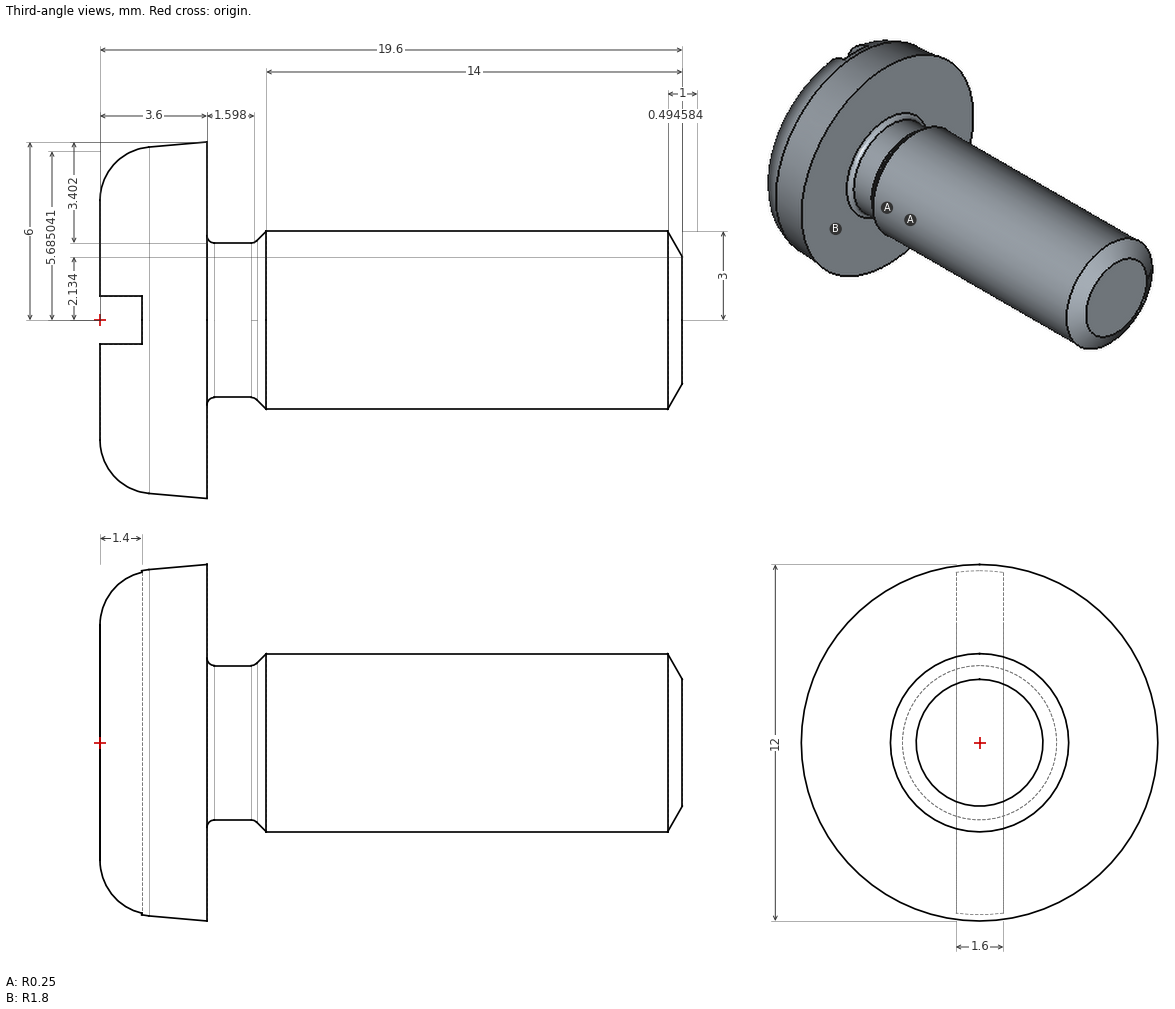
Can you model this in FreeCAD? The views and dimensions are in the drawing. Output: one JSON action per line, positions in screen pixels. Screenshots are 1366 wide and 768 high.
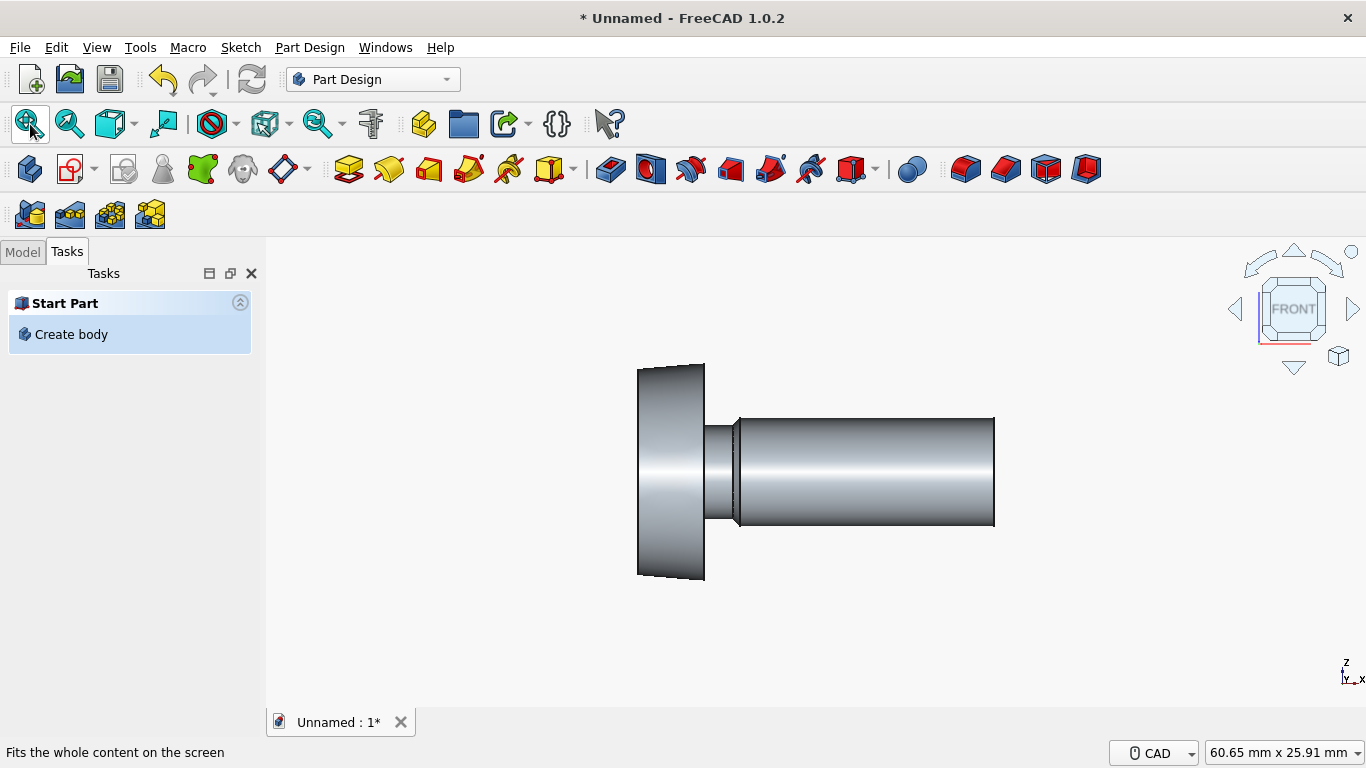
{"action": "key", "text": "3"}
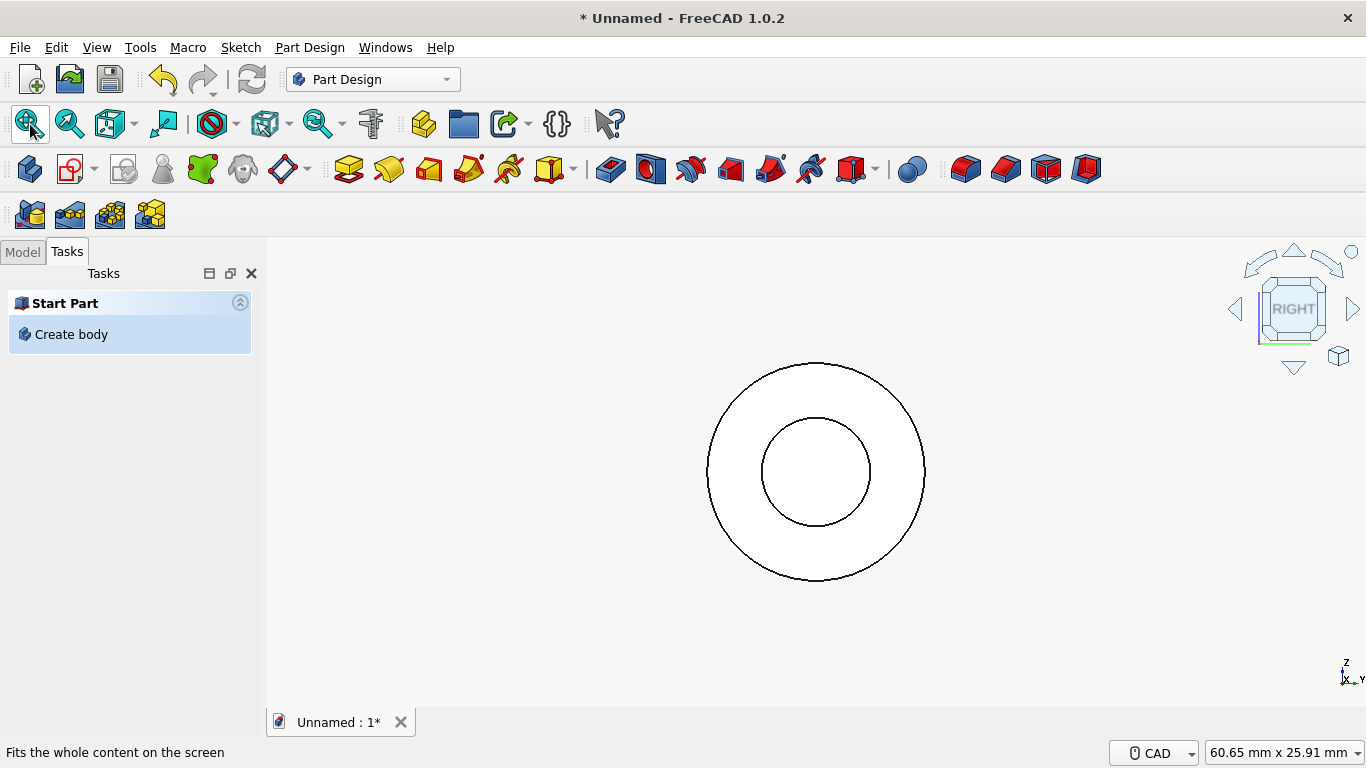
{"action": "key", "text": "5"}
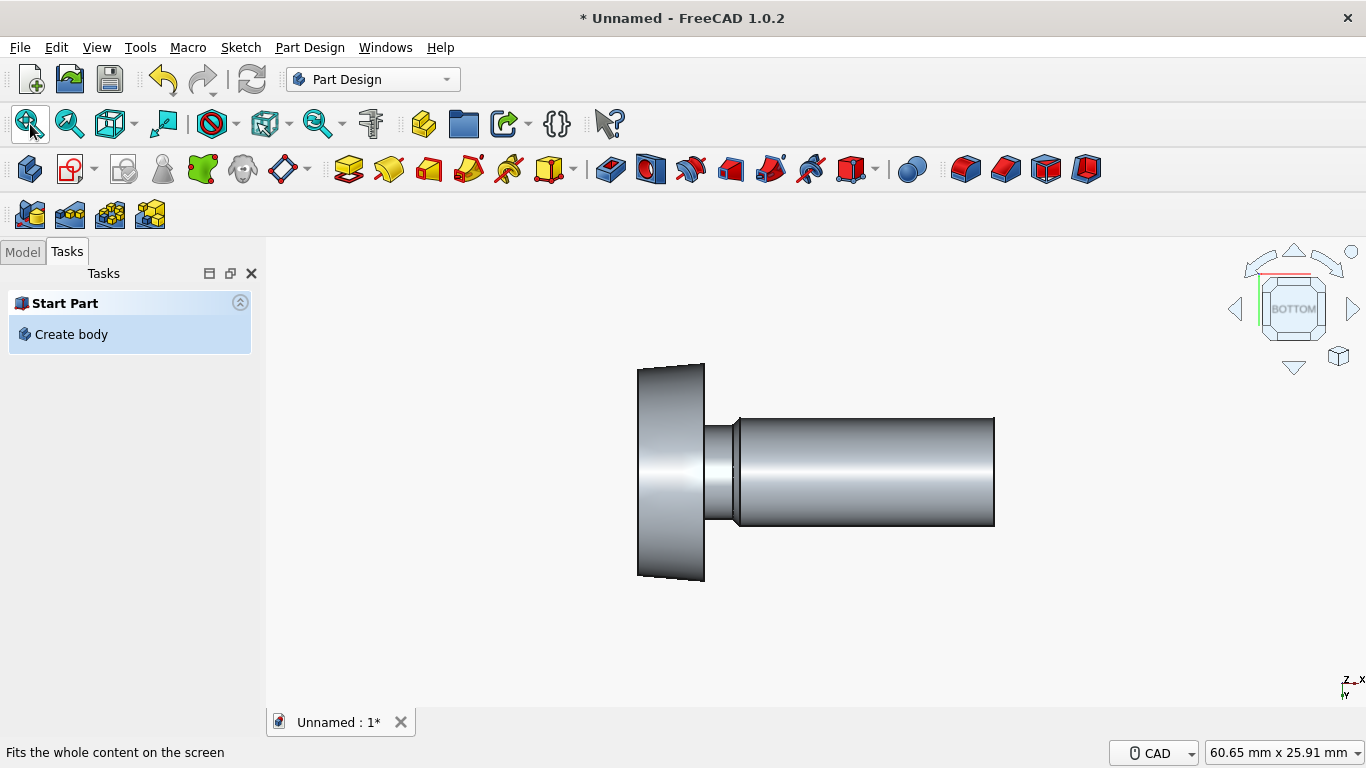
{"action": "key", "text": "4"}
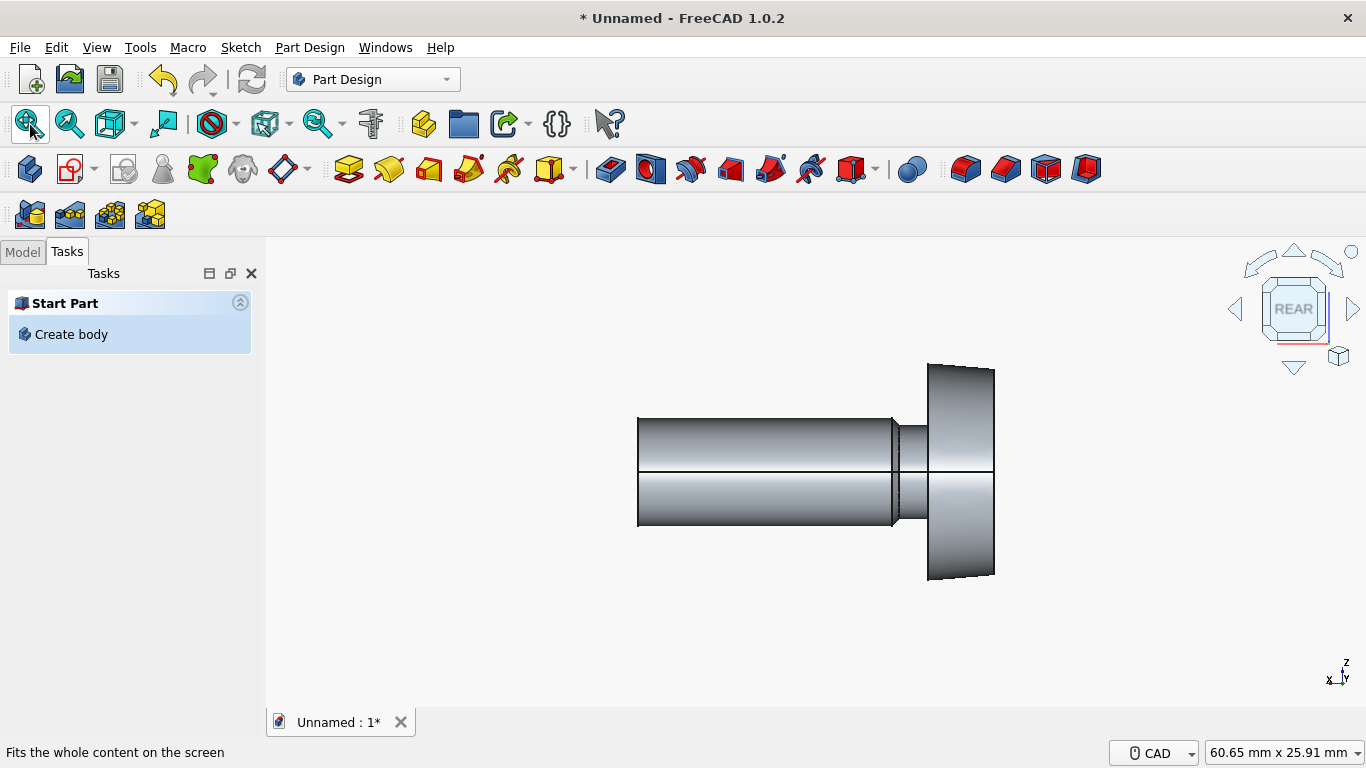
{"action": "key", "text": "6"}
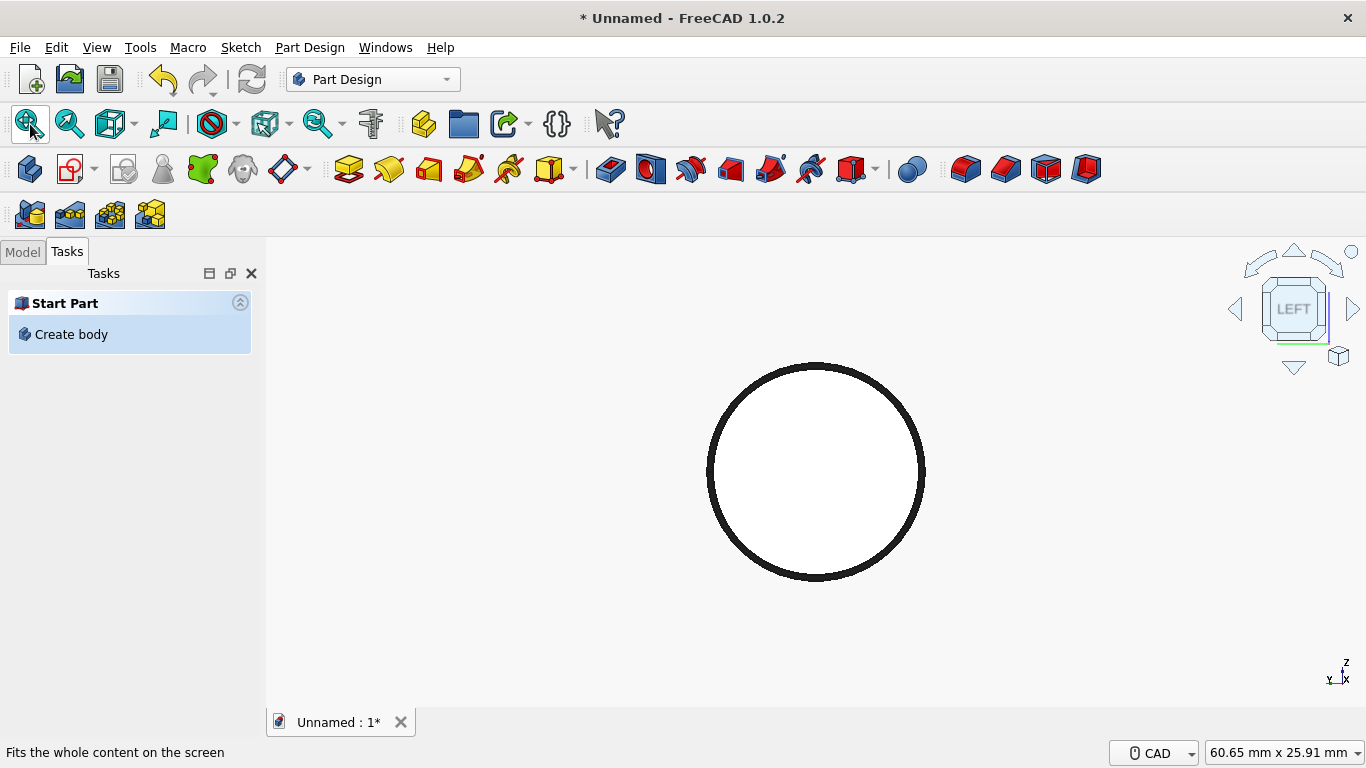
{"action": "key", "text": "v 3"}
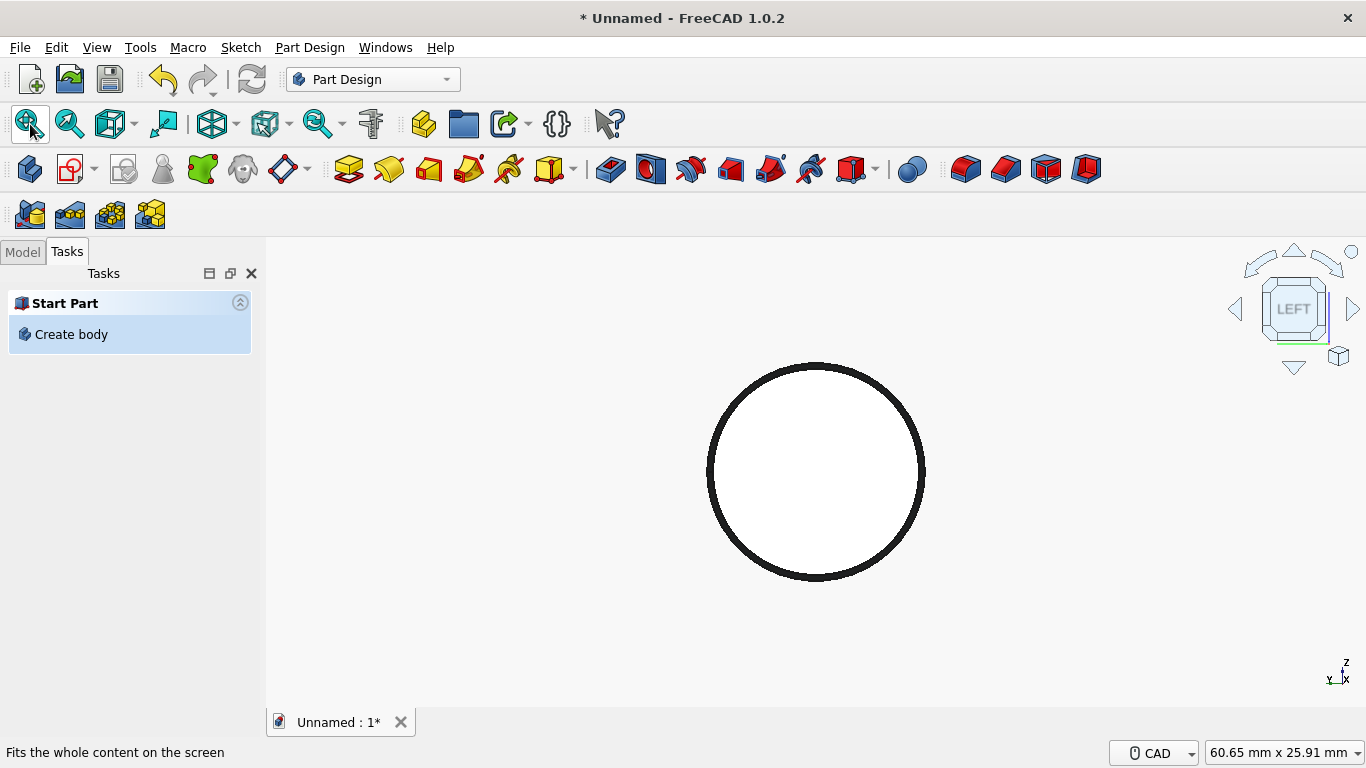
{"action": "key", "text": "0"}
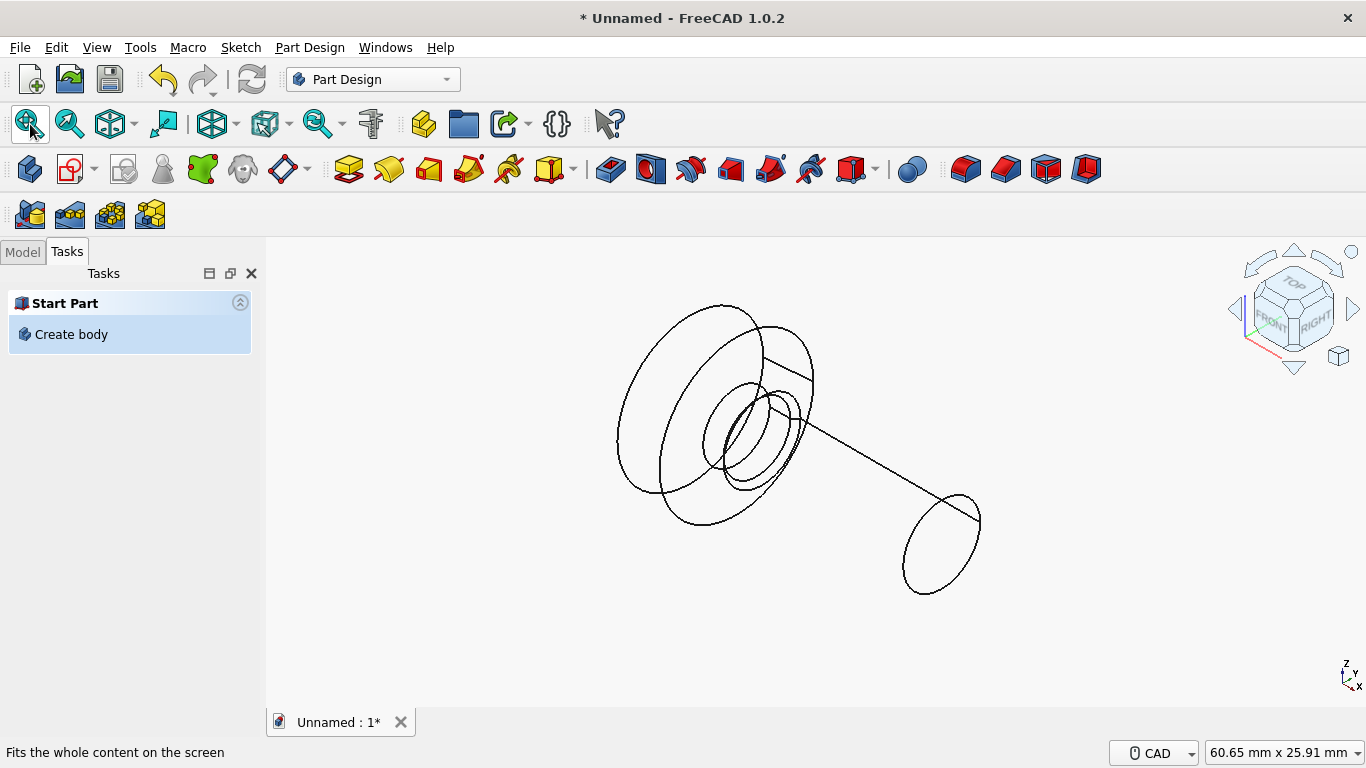
{"action": "left_click", "coordinate": [703, 444]}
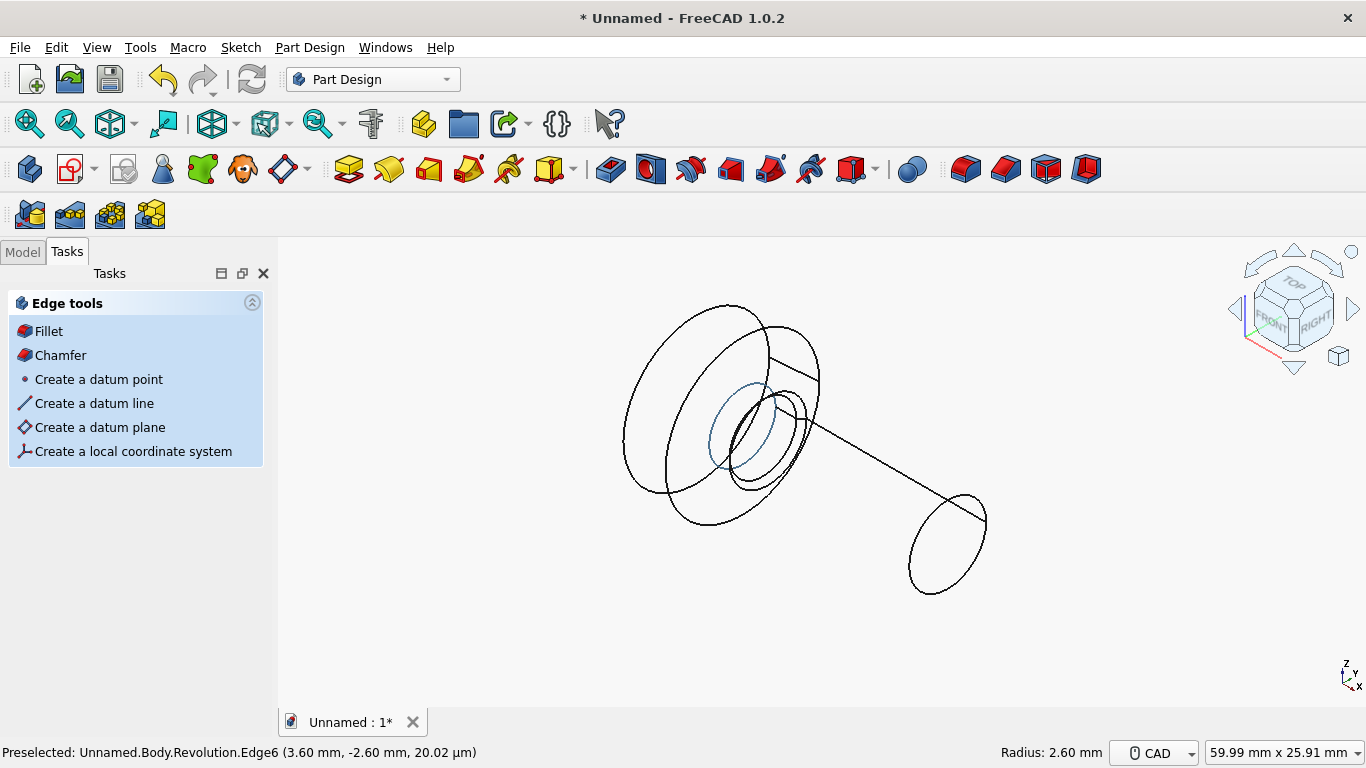
{"action": "left_click", "coordinate": [753, 479], "text": "ctrl"}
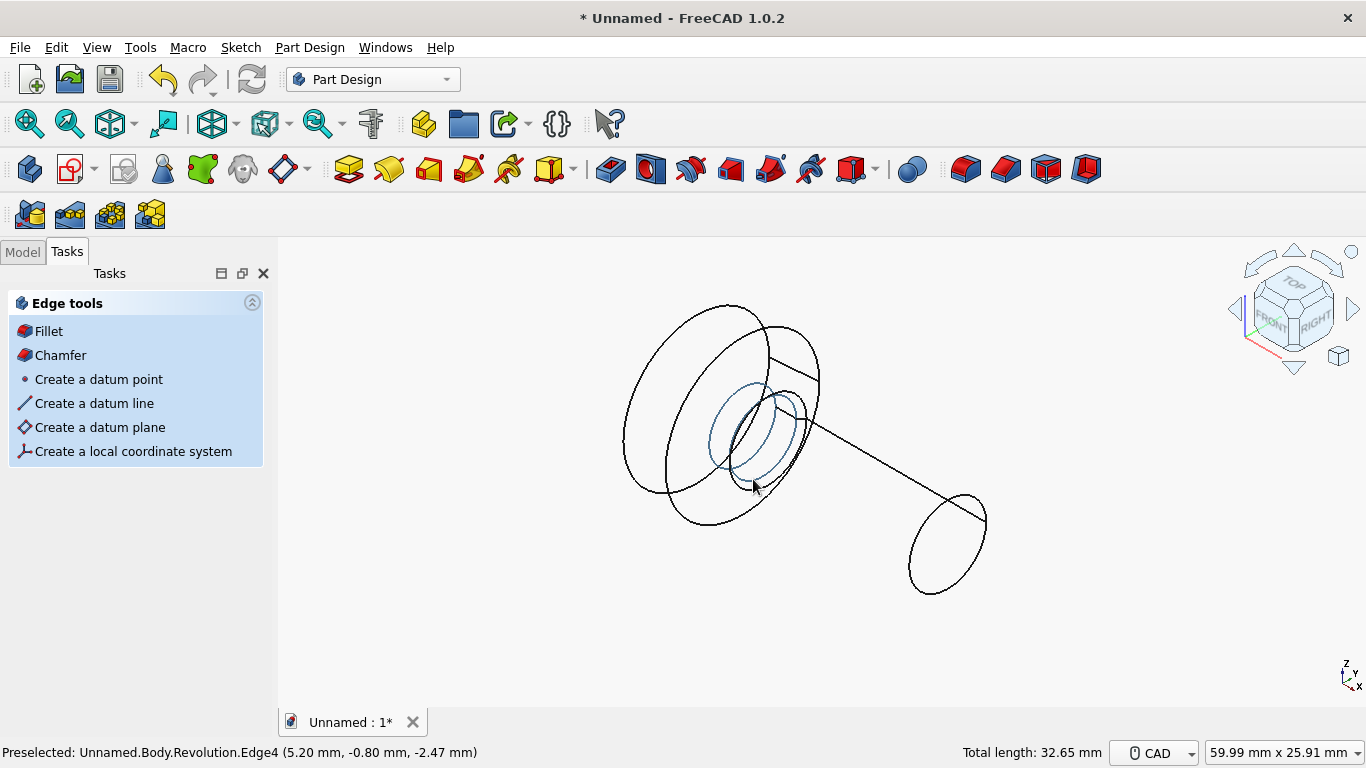
{"action": "key", "text": "v 1"}